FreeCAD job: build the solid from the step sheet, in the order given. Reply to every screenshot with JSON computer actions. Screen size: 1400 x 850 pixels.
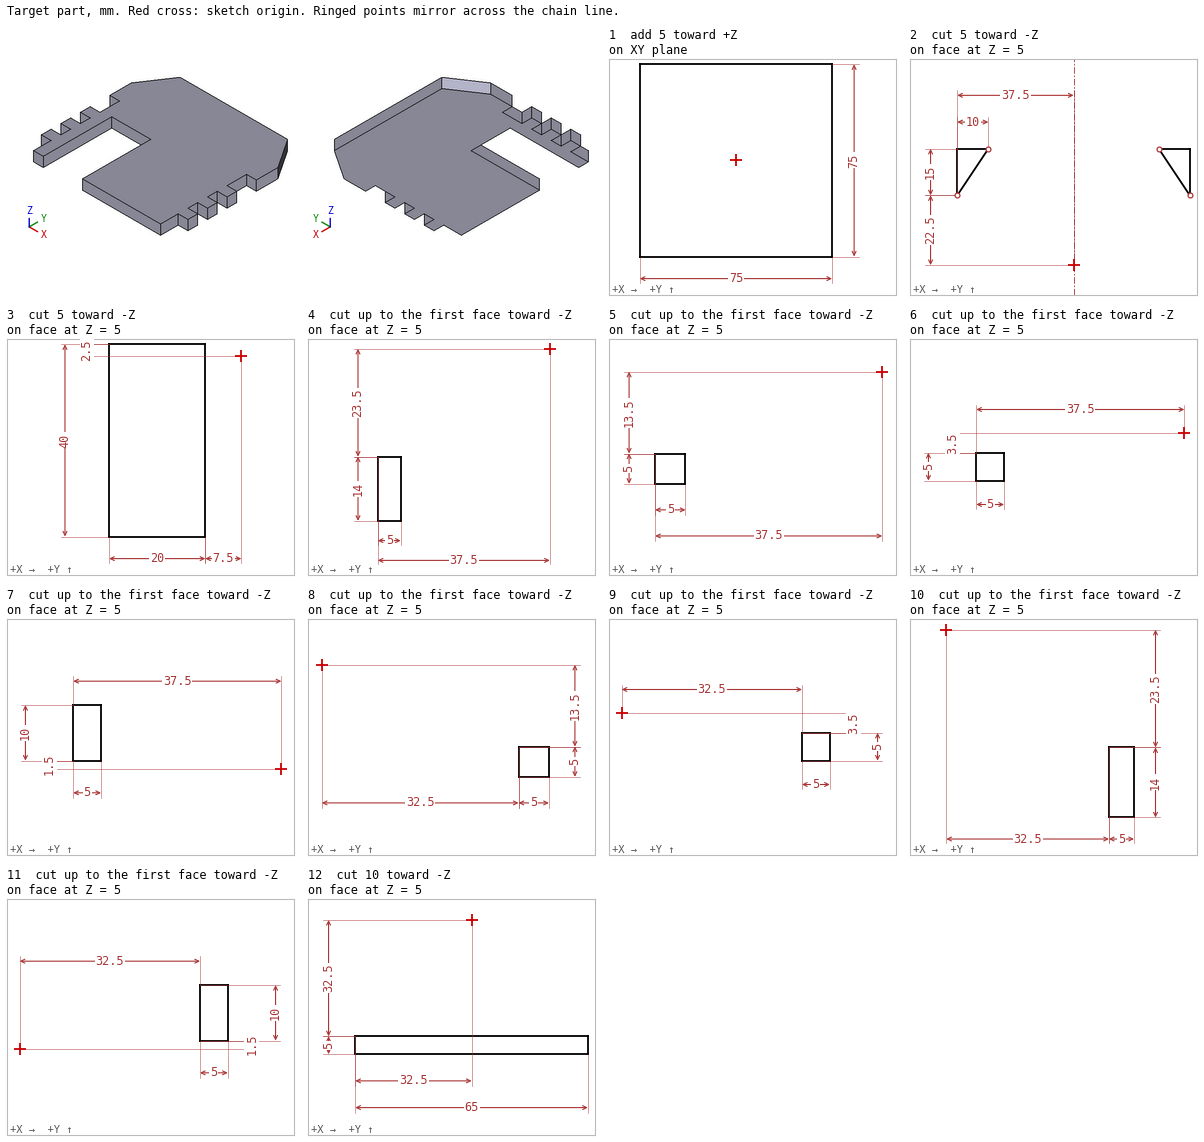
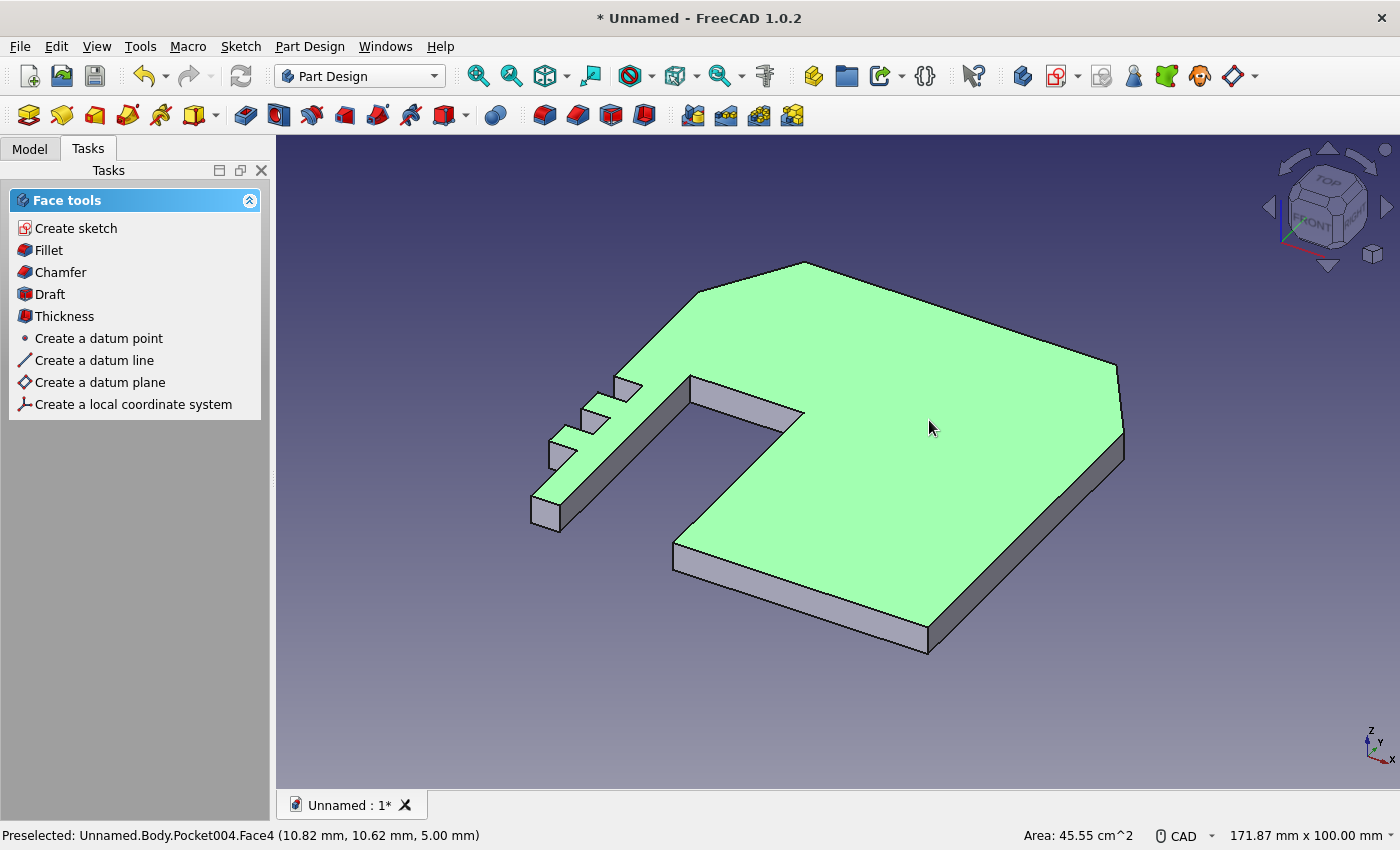
{"action": "left_click", "coordinate": [1056, 76]}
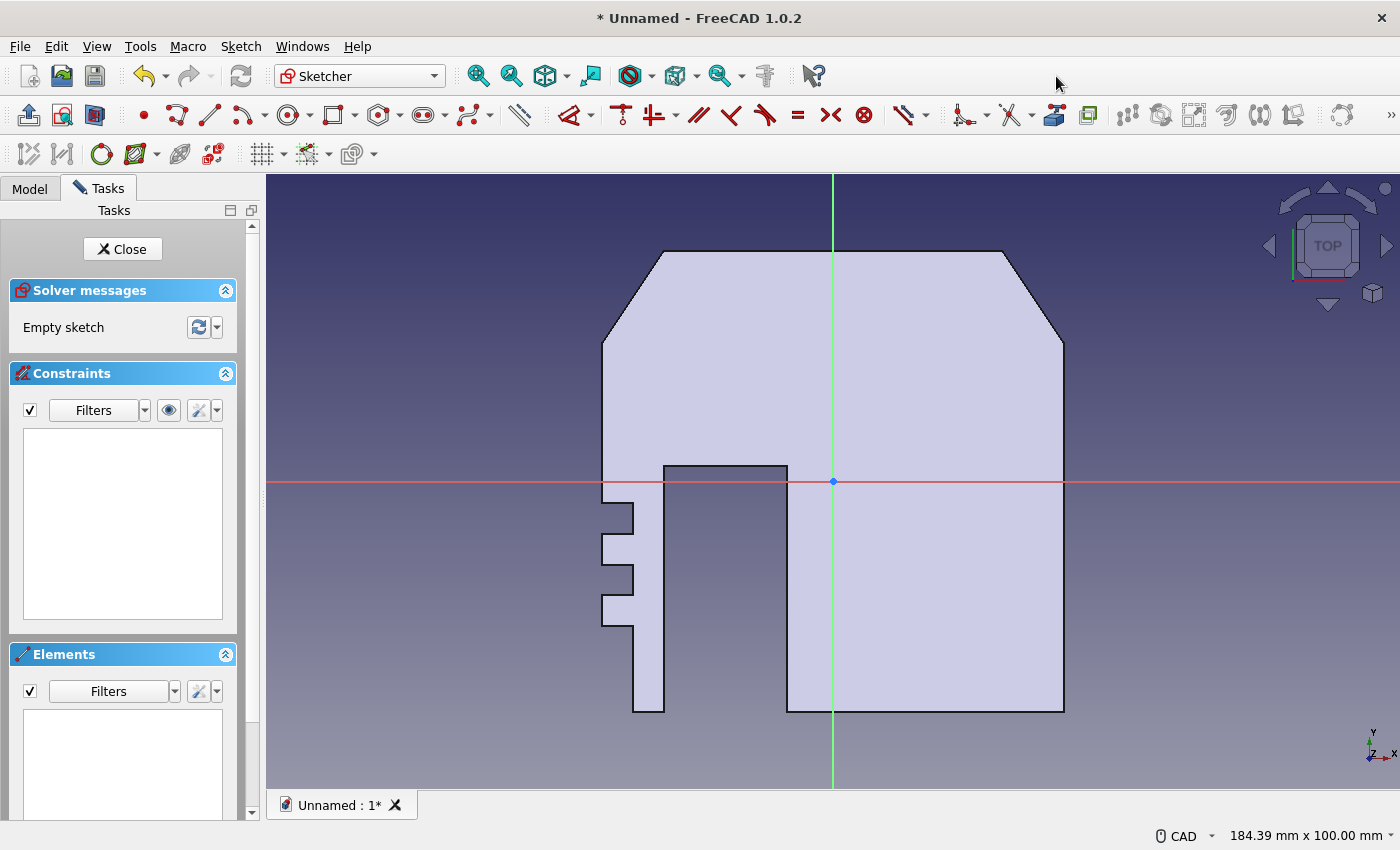
{"action": "scroll", "coordinate": [589, 434], "scroll_direction": "up", "scroll_amount": 9}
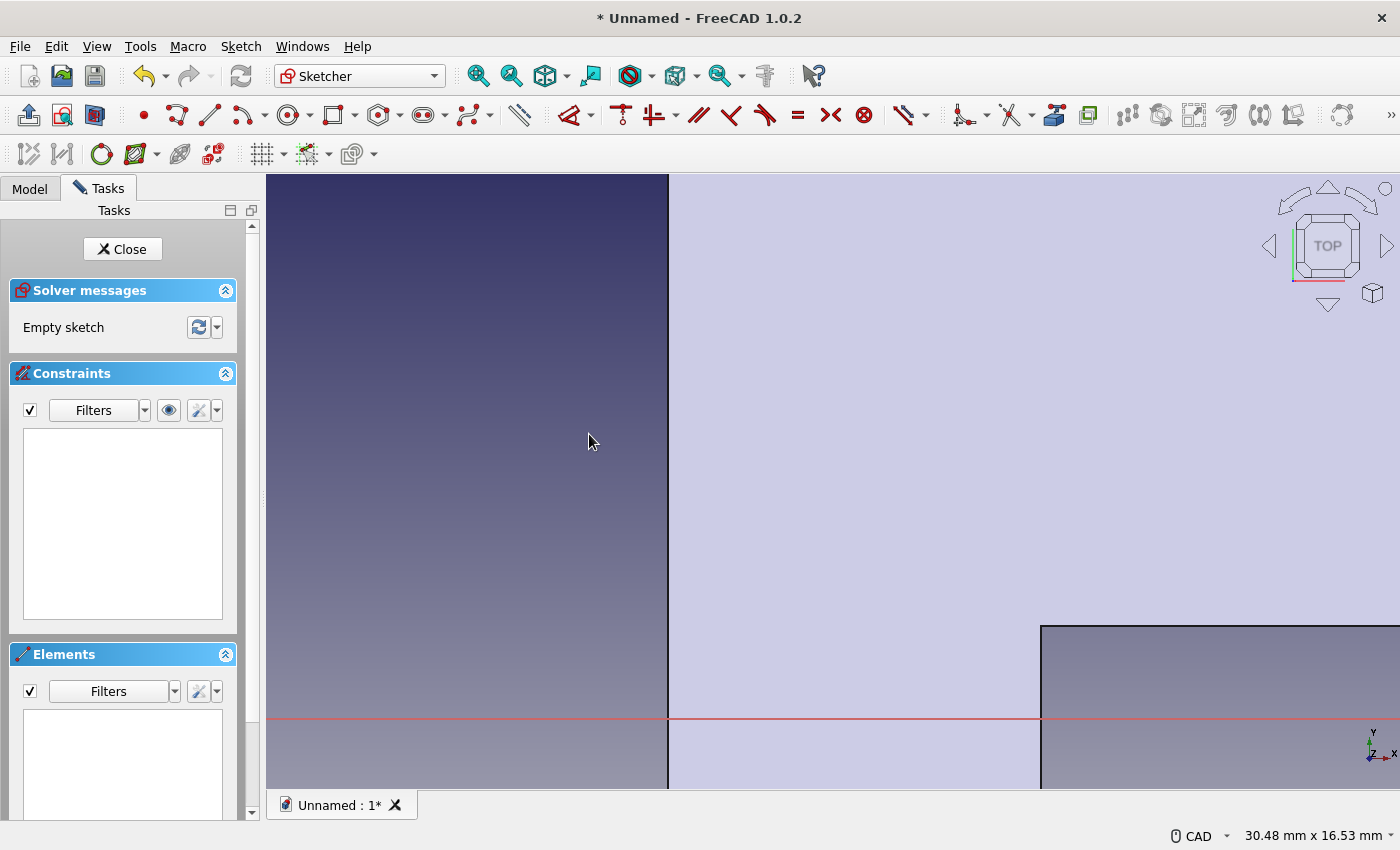
{"action": "left_click", "coordinate": [332, 116]}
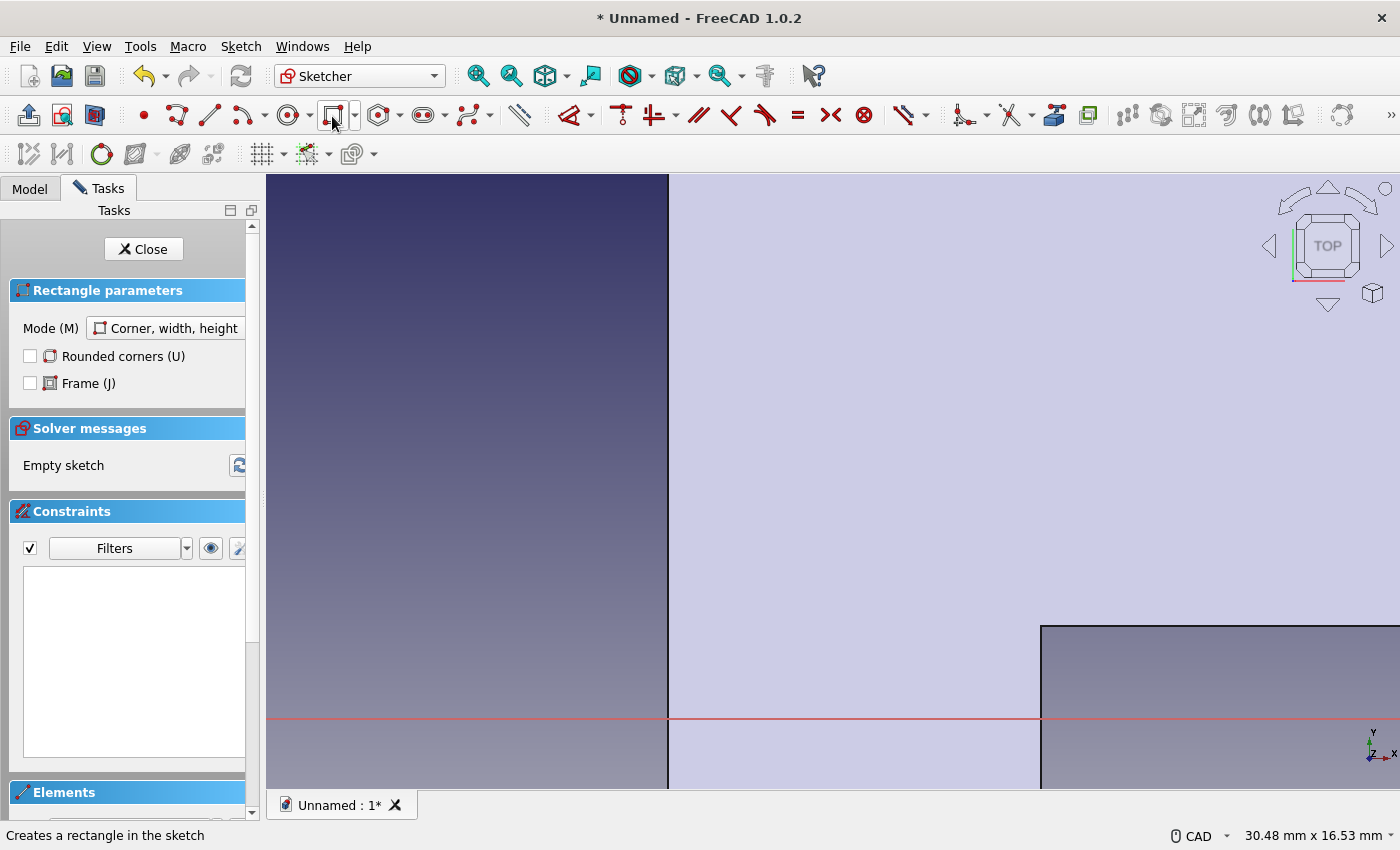
{"action": "left_click", "coordinate": [668, 291]}
{"action": "left_click", "coordinate": [855, 663]}
{"action": "key", "text": "Escape"}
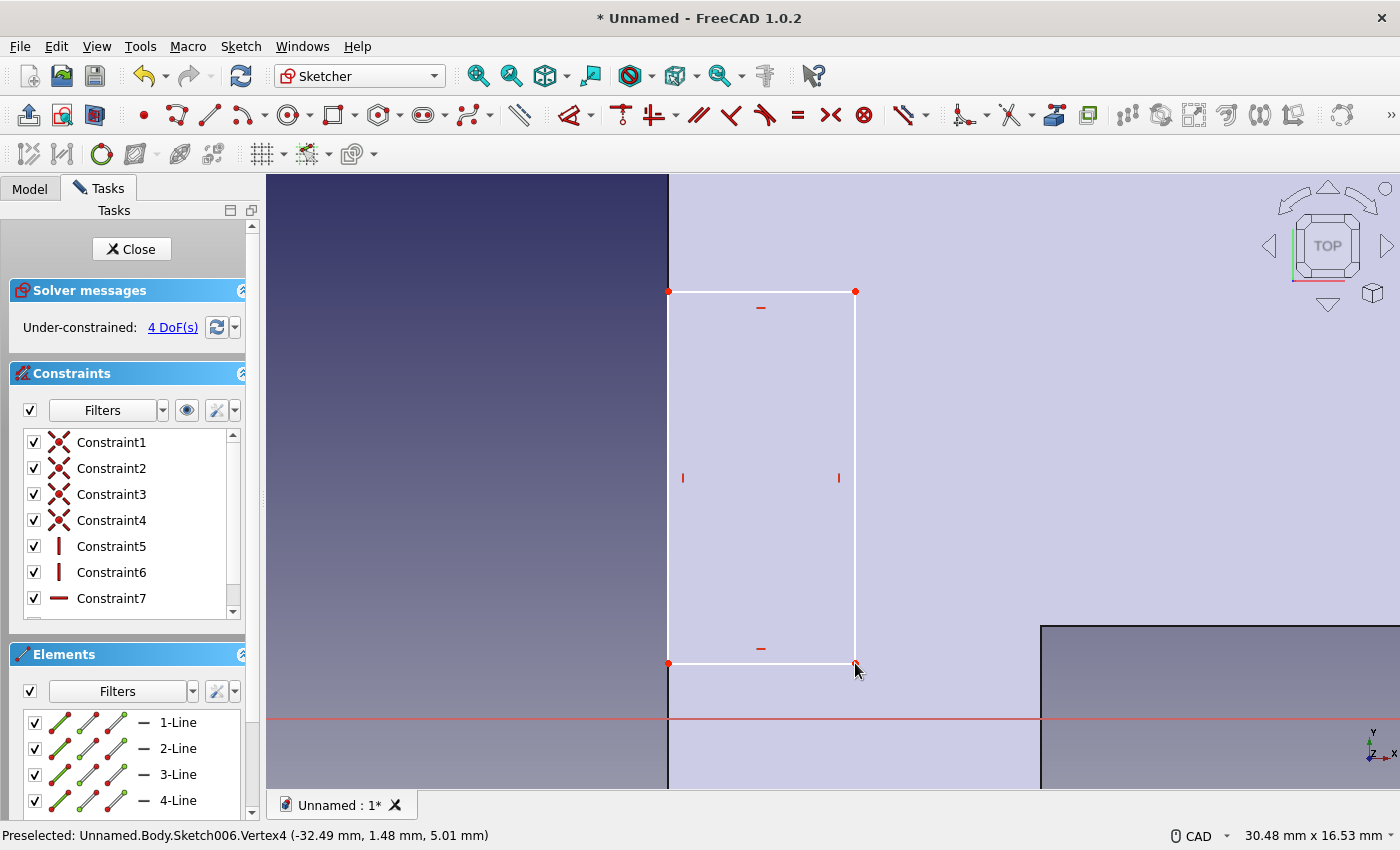
{"action": "left_click", "coordinate": [568, 116]}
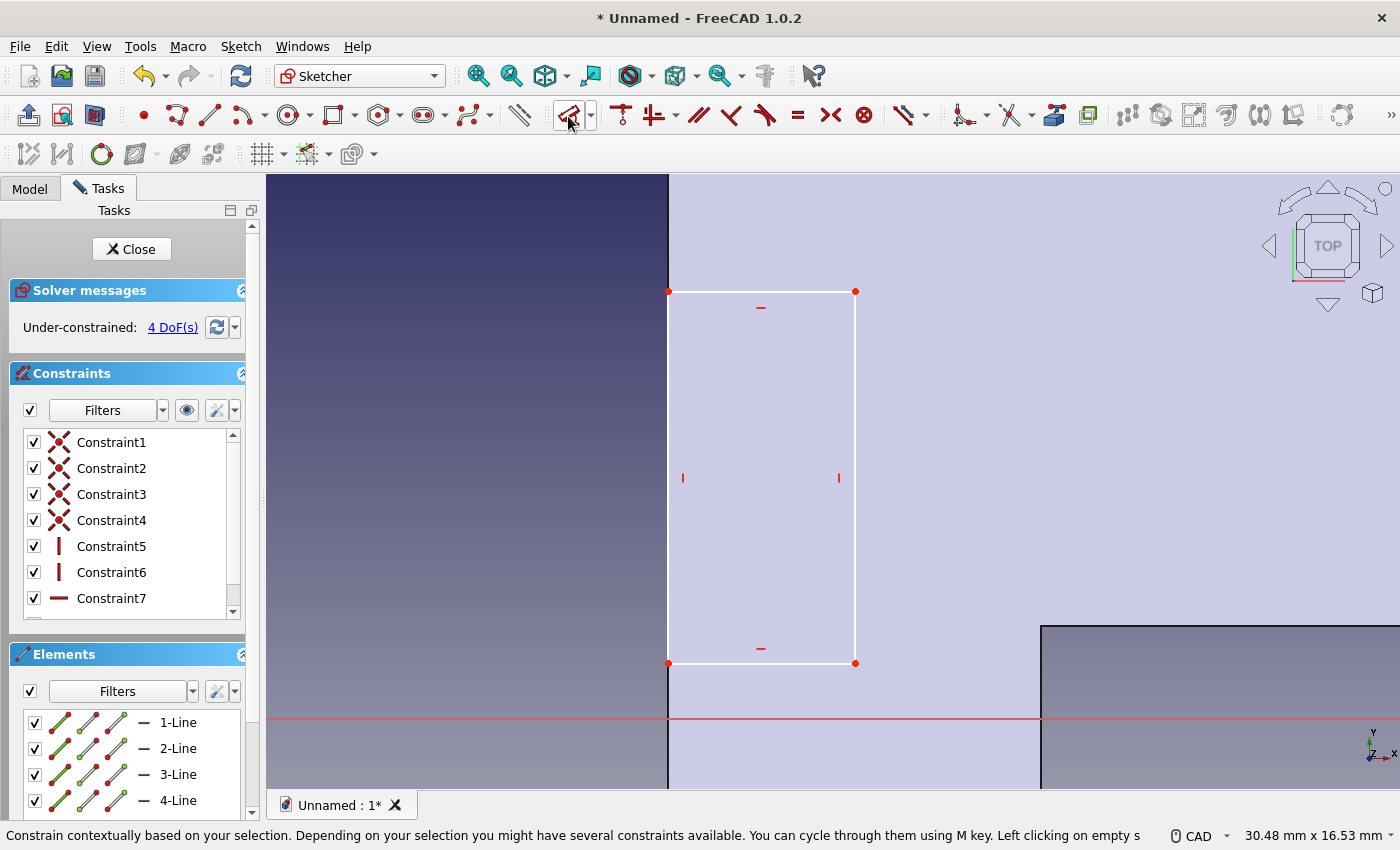
{"action": "left_click", "coordinate": [724, 664]}
{"action": "left_click", "coordinate": [761, 698]}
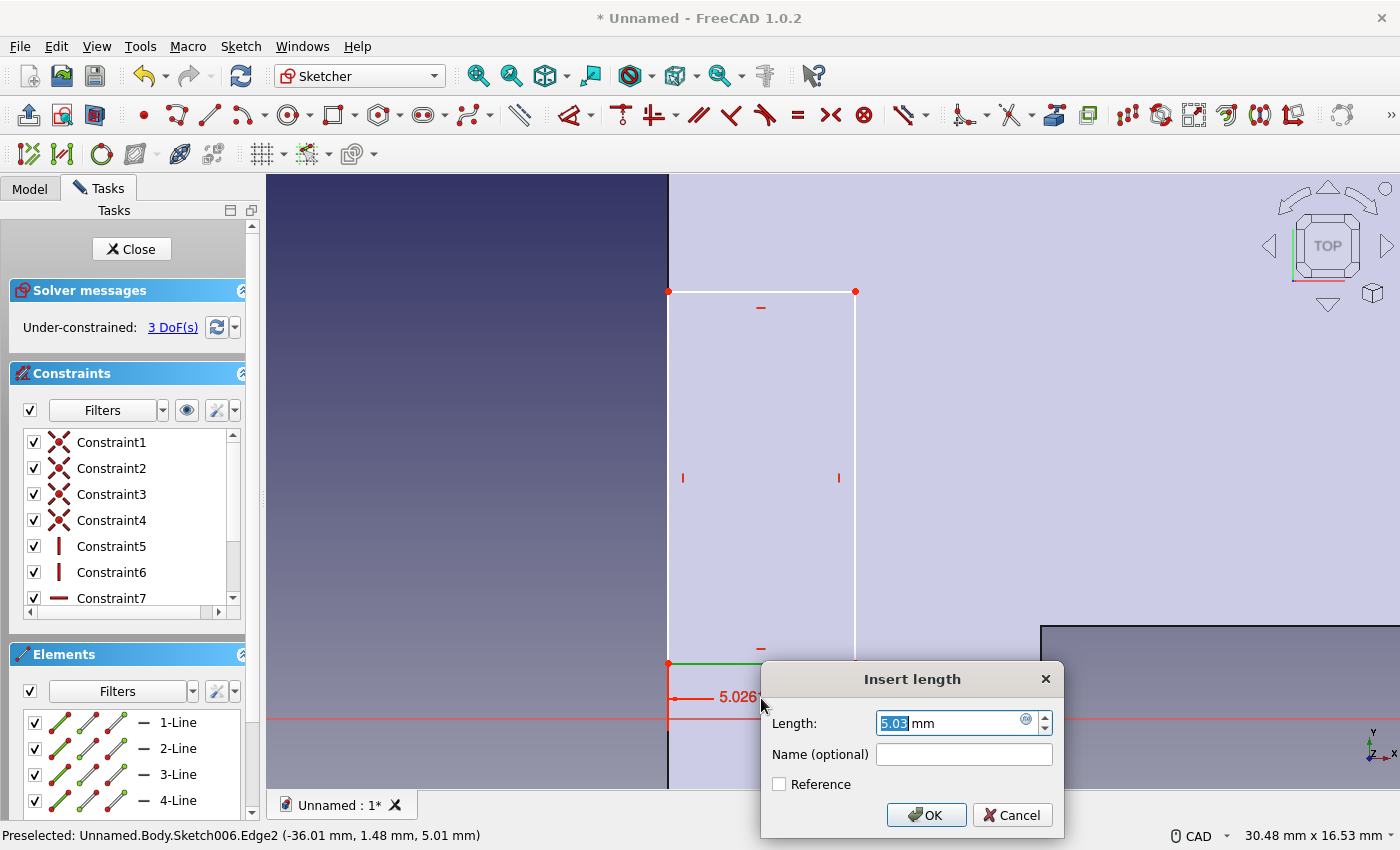
{"action": "type", "text": "5"}
{"action": "key", "text": "Return"}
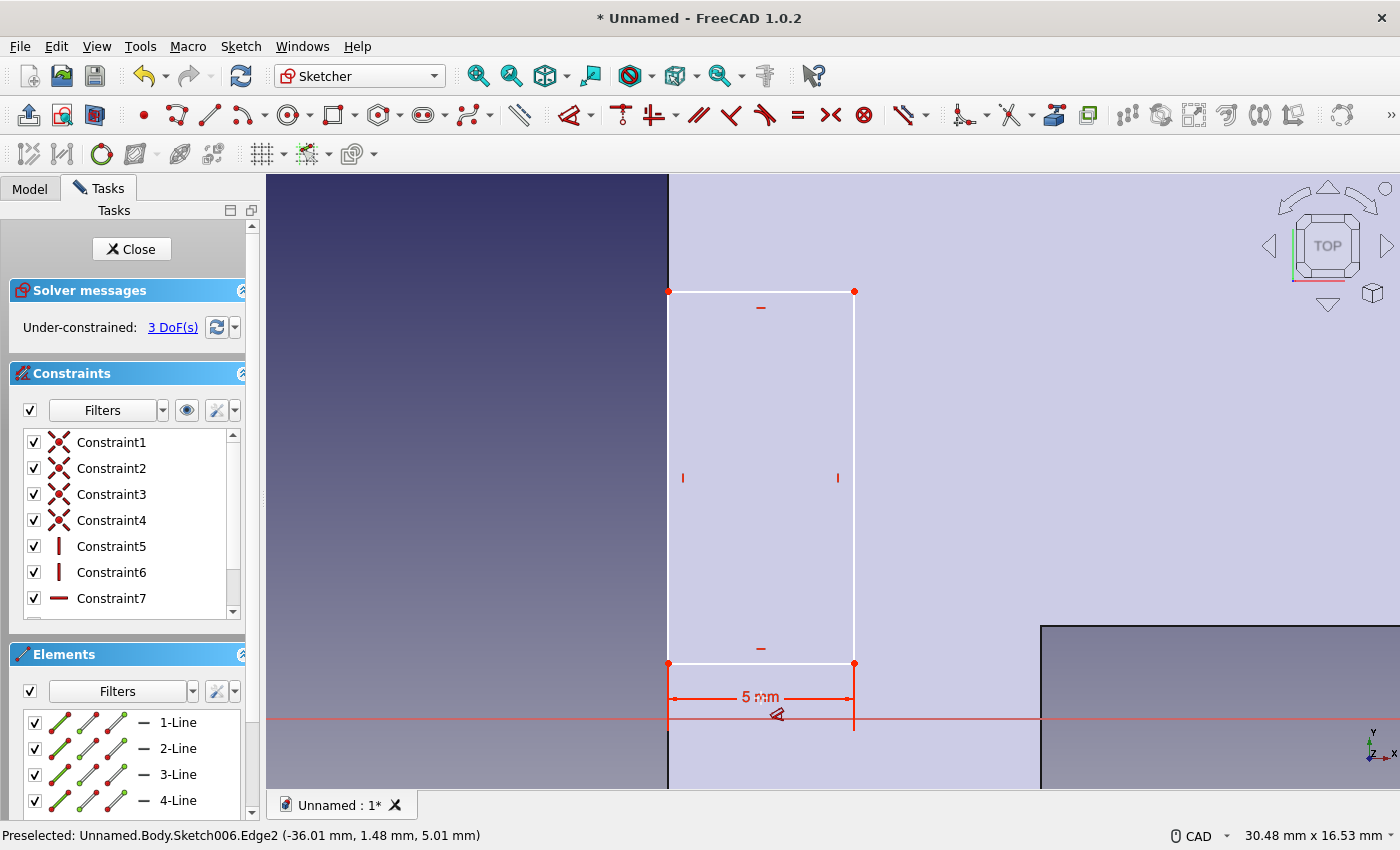
{"action": "left_click", "coordinate": [668, 404]}
{"action": "left_click", "coordinate": [634, 478]}